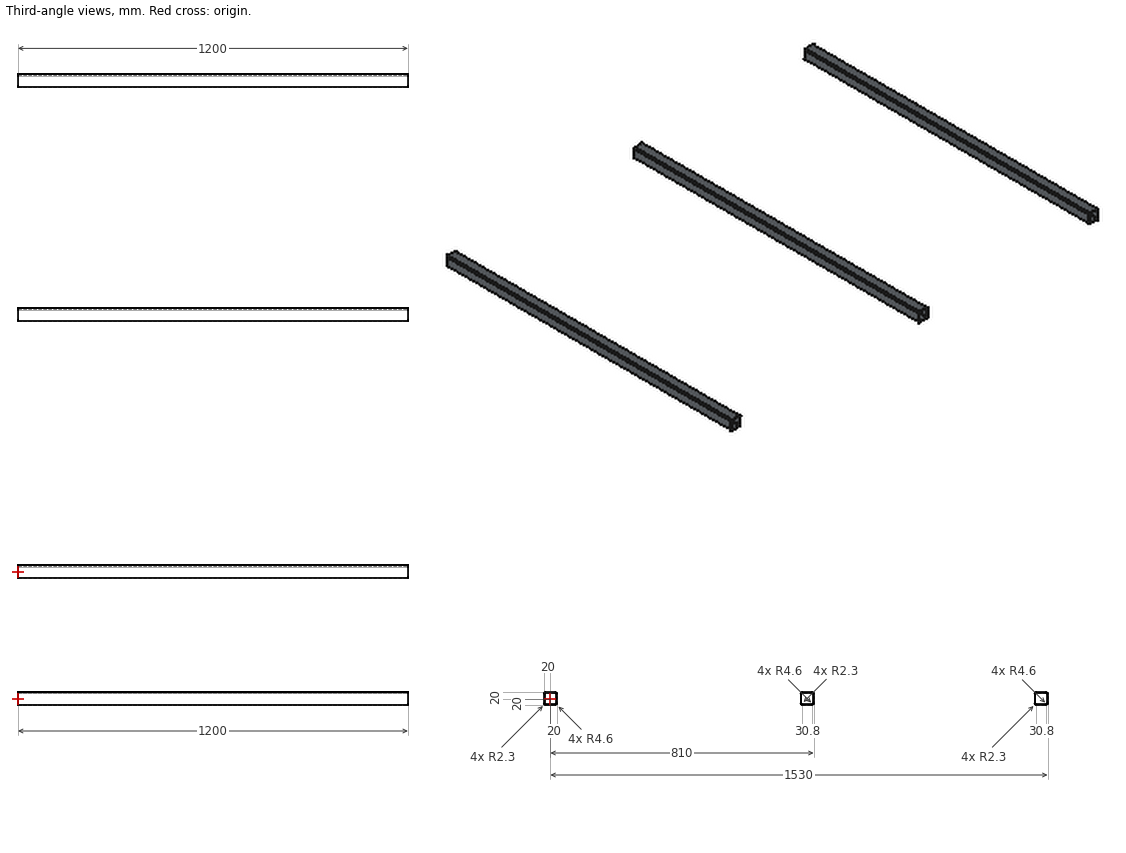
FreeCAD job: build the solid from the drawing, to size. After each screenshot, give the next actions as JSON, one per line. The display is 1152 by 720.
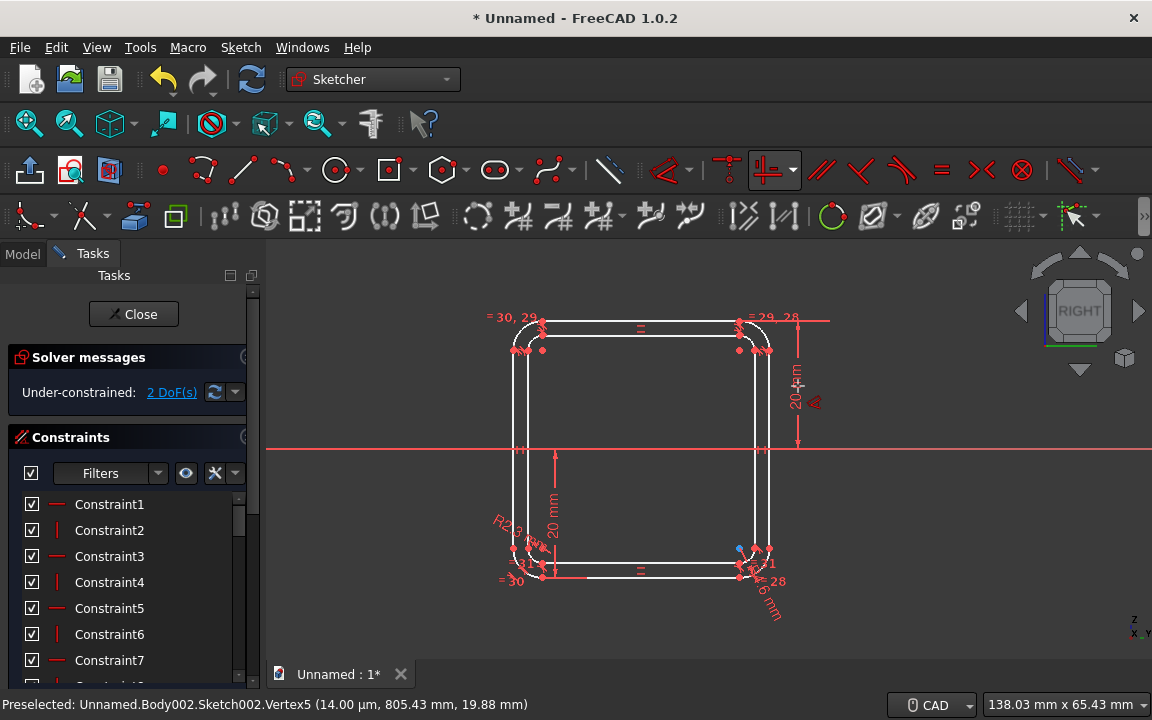
{"action": "left_click", "coordinate": [602, 578]}
{"action": "left_click", "coordinate": [641, 612]}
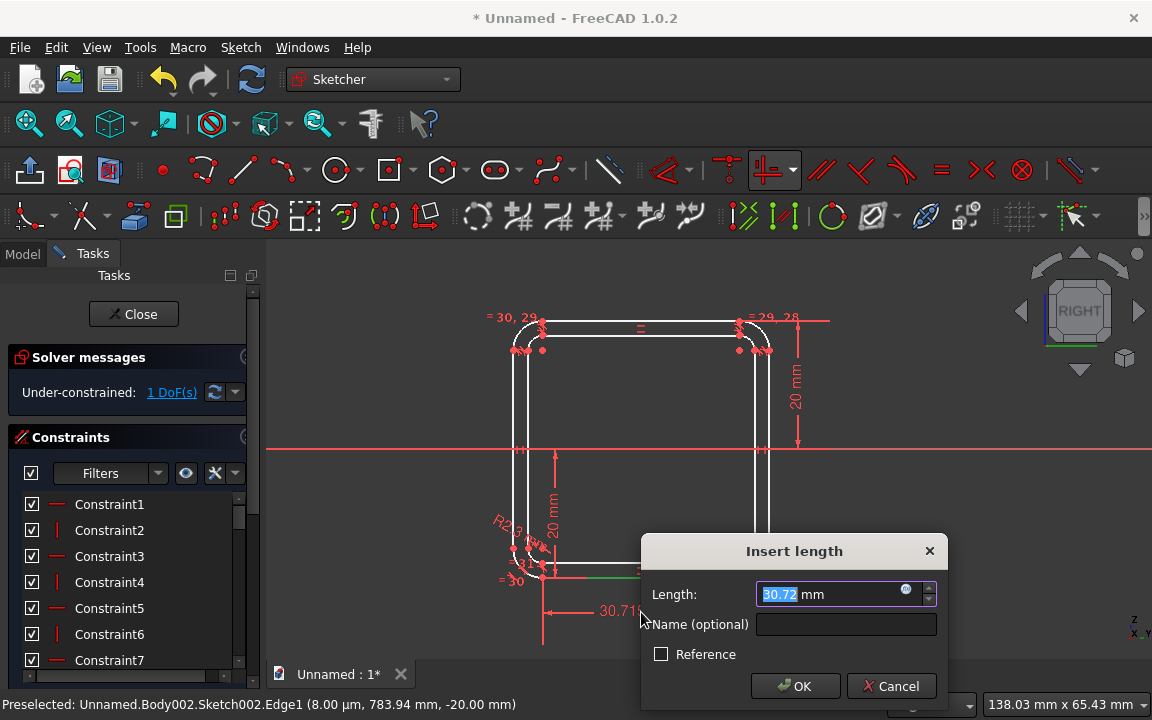
{"action": "type", "text": "30.8"}
{"action": "key", "text": "Return"}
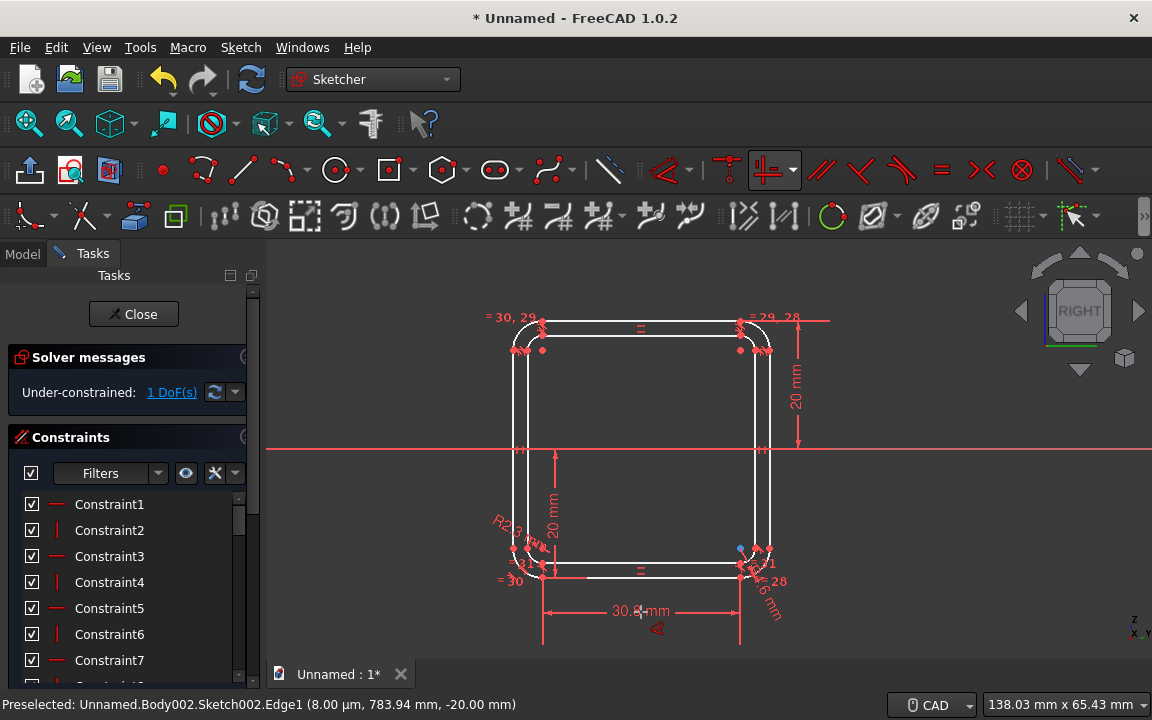
{"action": "left_click", "coordinate": [770, 548]}
{"action": "left_click", "coordinate": [422, 582]}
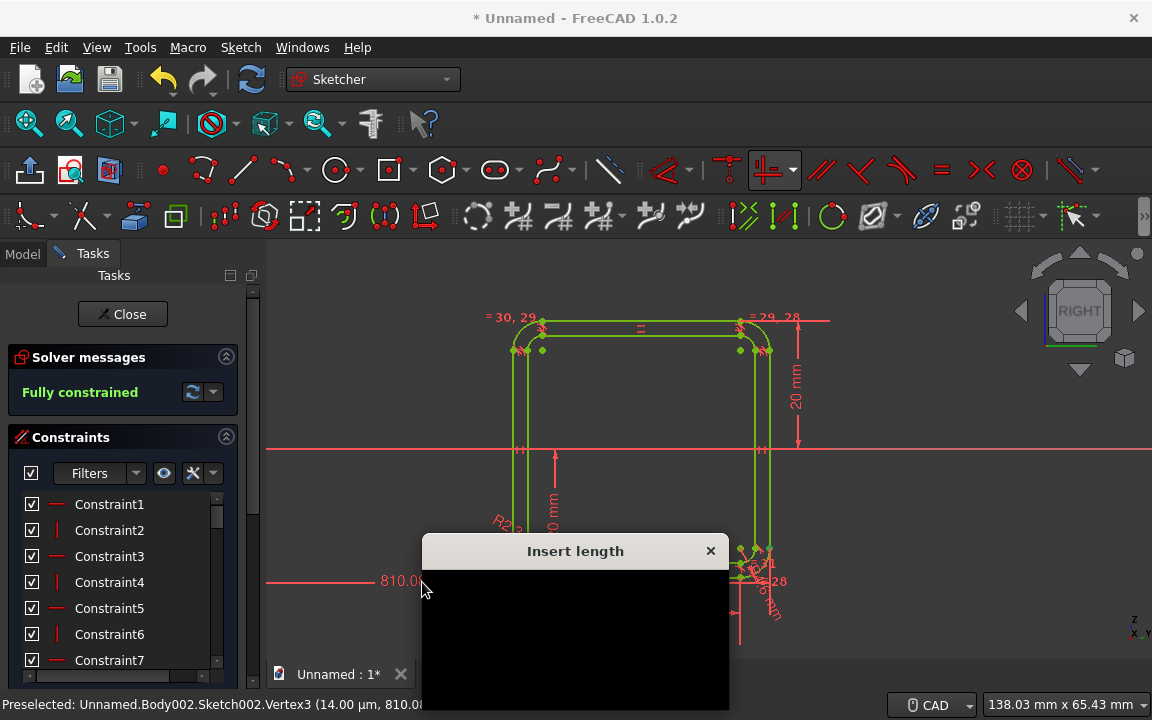
{"action": "type", "text": "810"}
{"action": "key", "text": "Return"}
{"action": "key", "text": "Escape"}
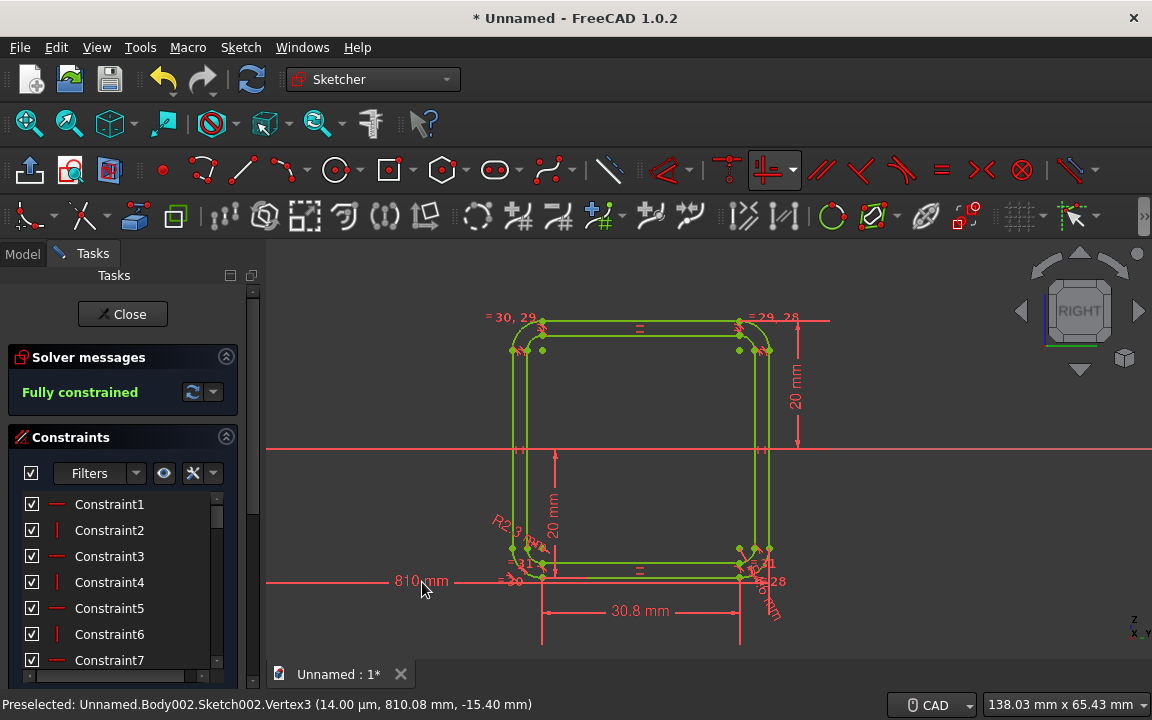
{"action": "left_click", "coordinate": [123, 314]}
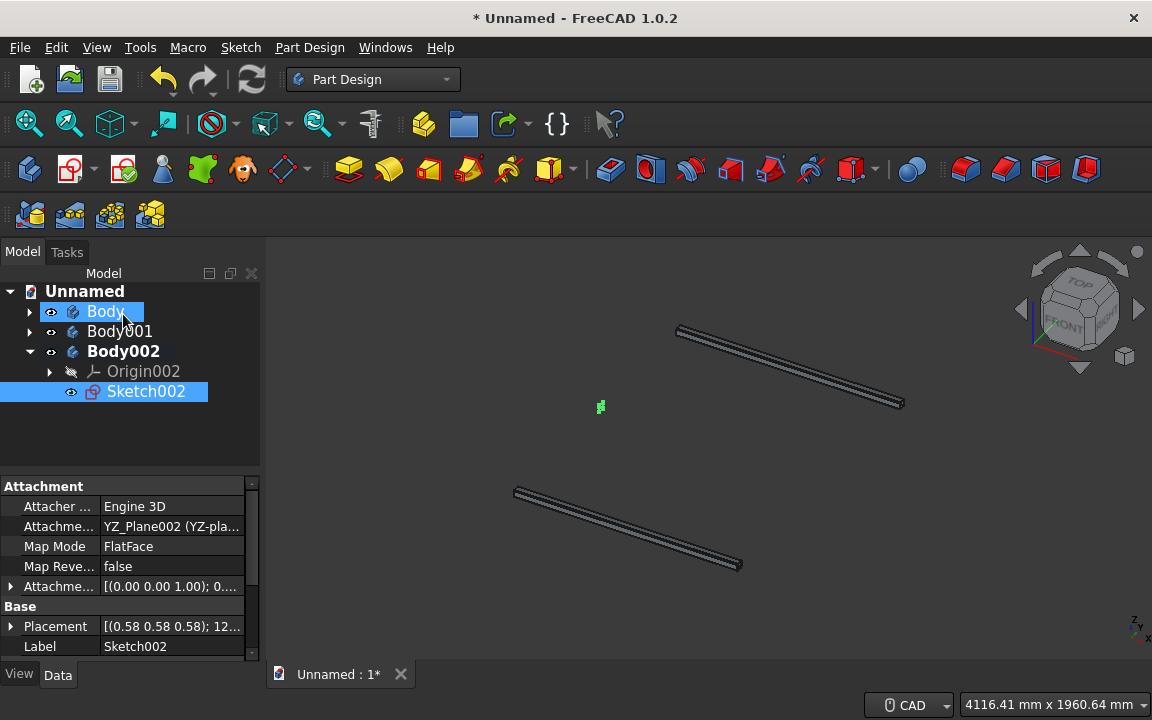
{"action": "left_click", "coordinate": [350, 170]}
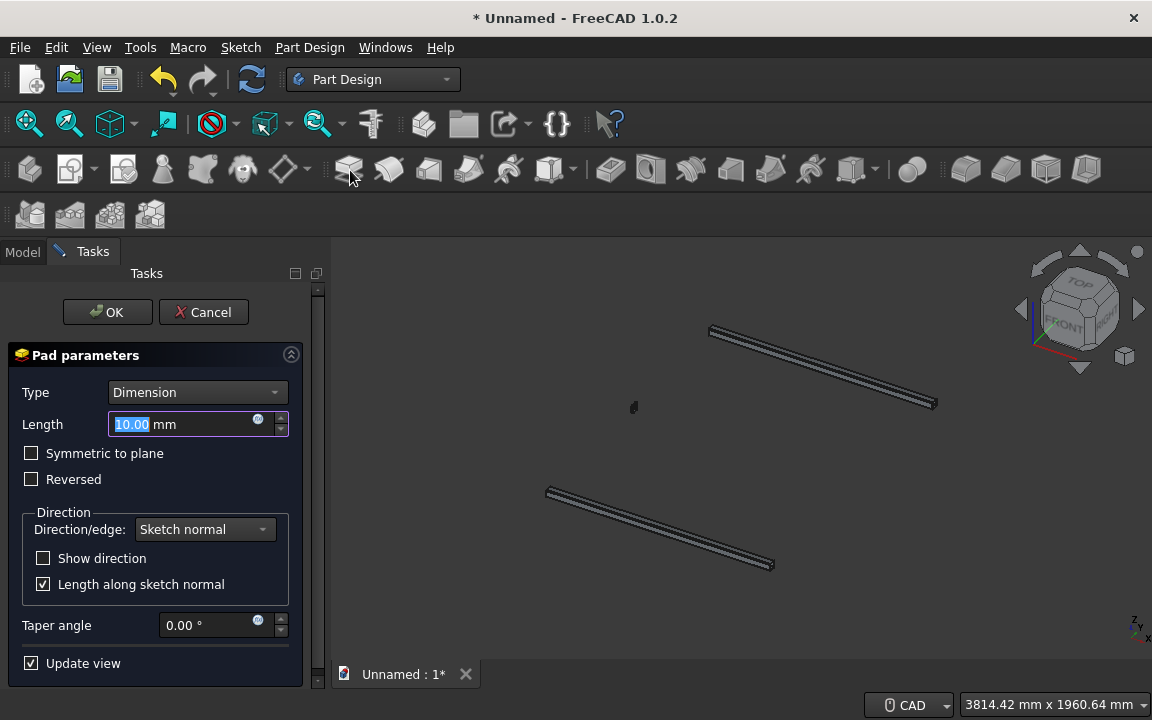
{"action": "type", "text": "1200"}
{"action": "key", "text": "Tab"}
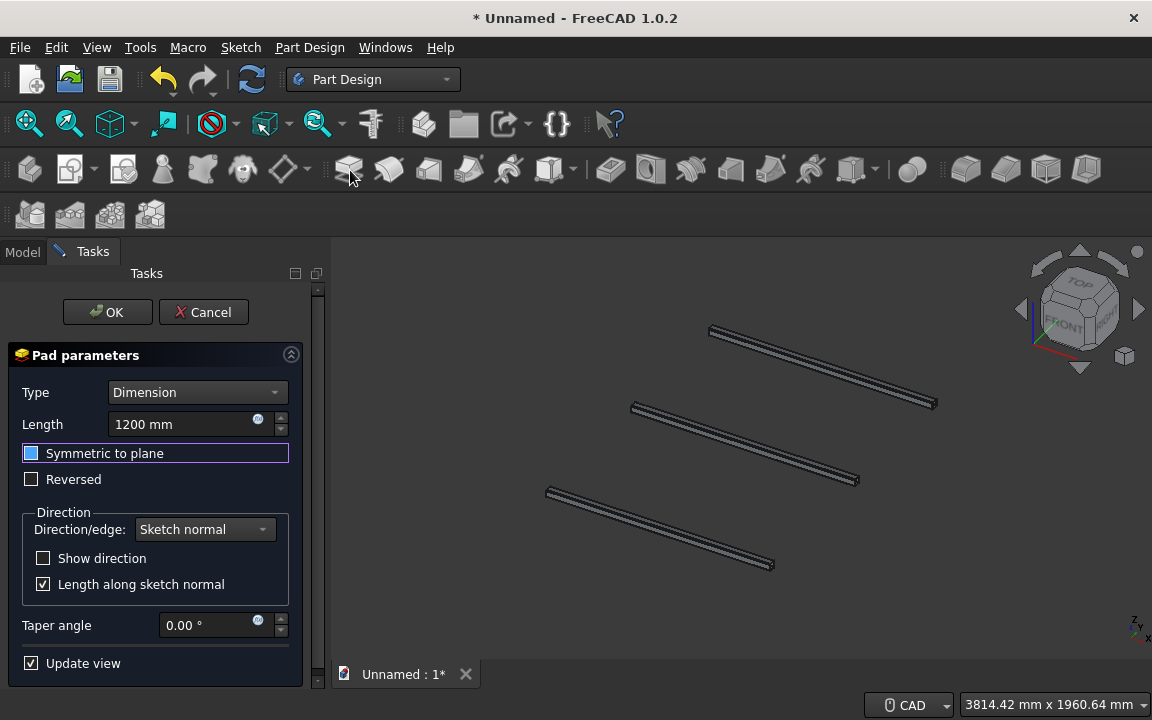
{"action": "left_click", "coordinate": [108, 312]}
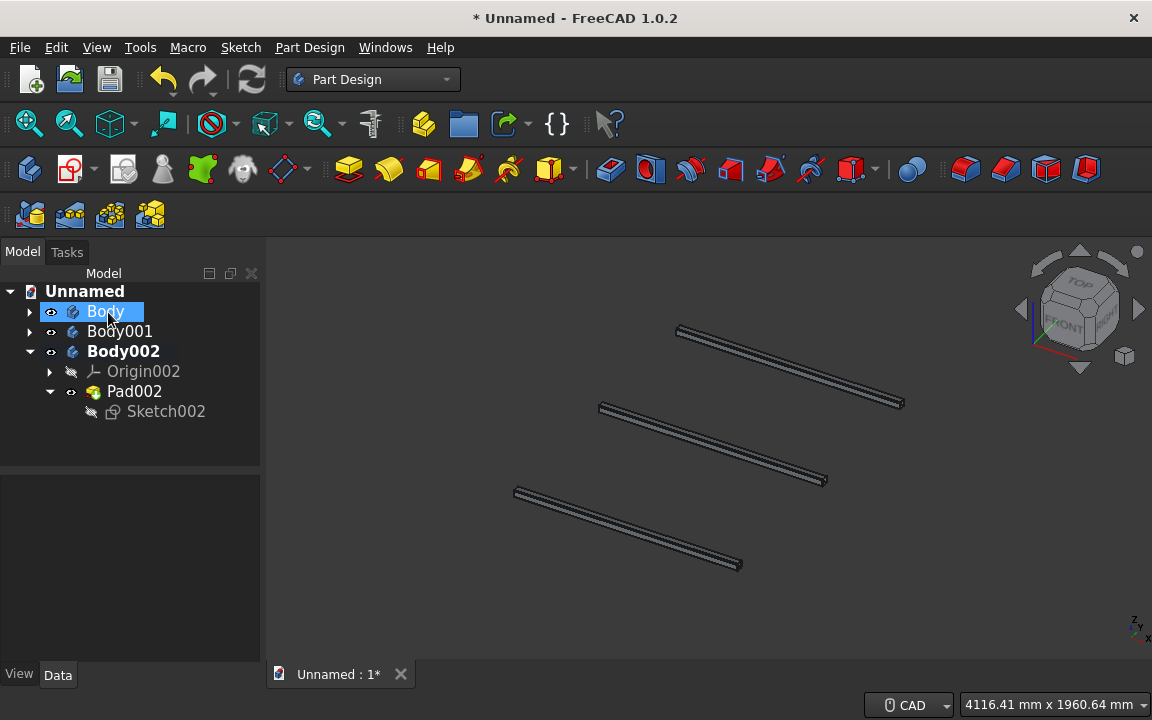
{"action": "key", "text": "0"}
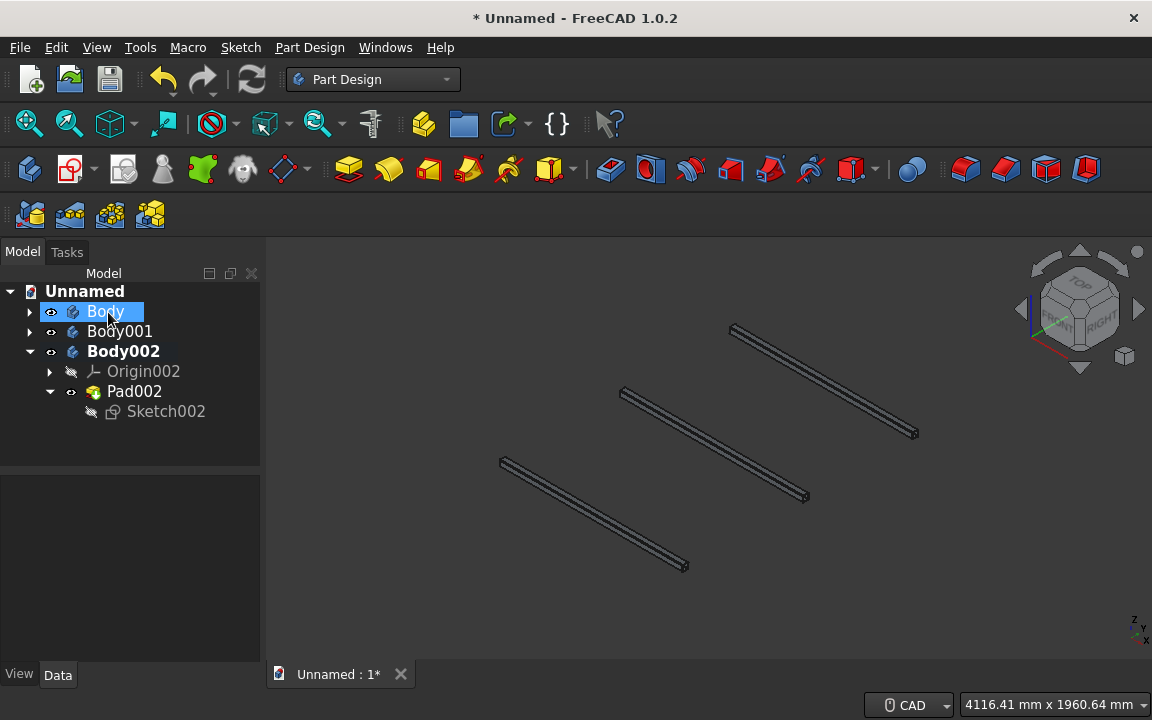
{"action": "key", "text": "v f"}